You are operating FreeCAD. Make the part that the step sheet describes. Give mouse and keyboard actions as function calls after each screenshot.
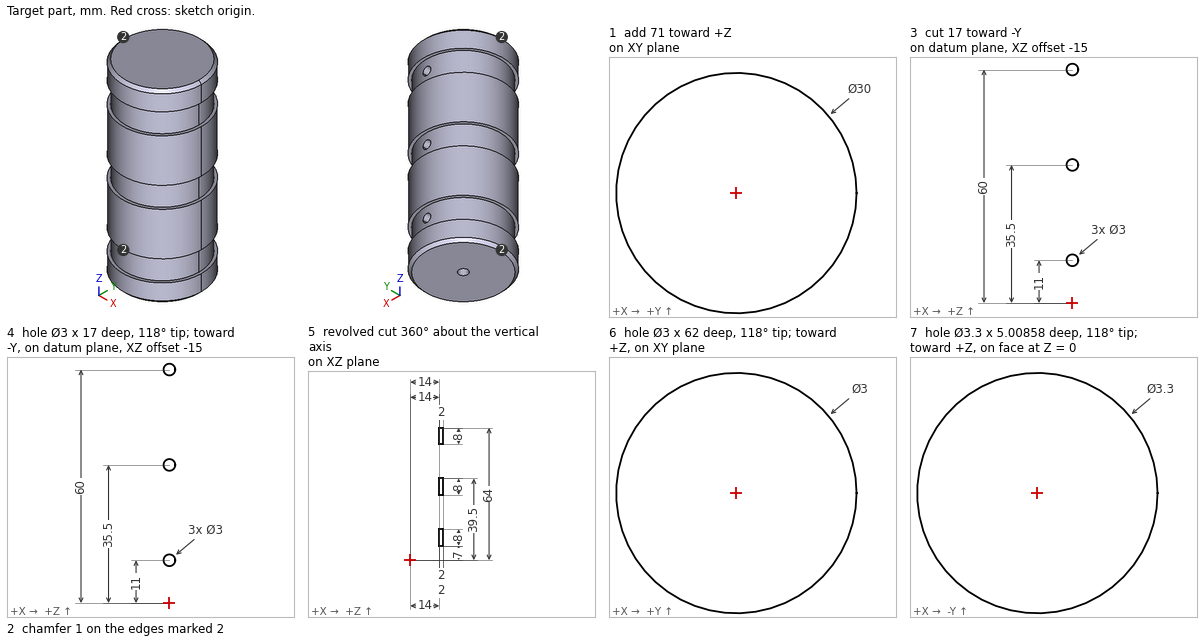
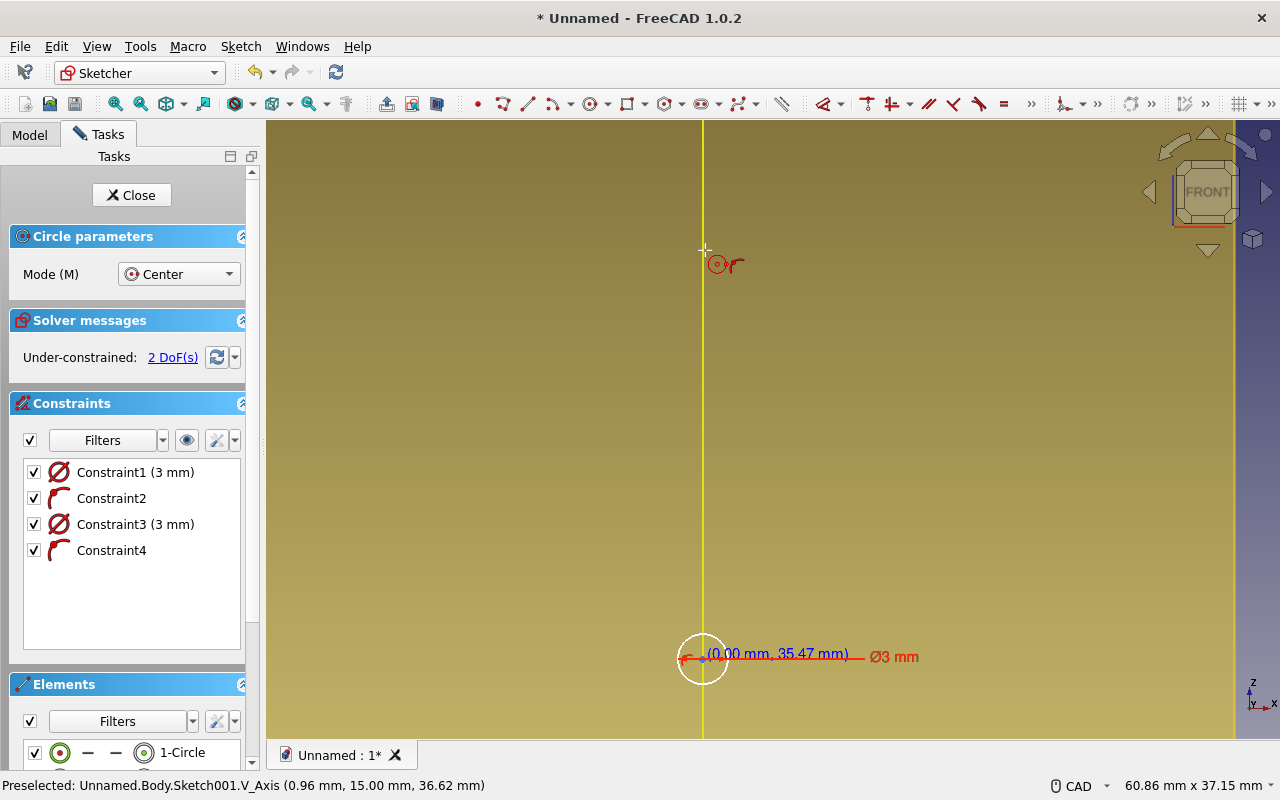
click(703, 250)
move(721, 233)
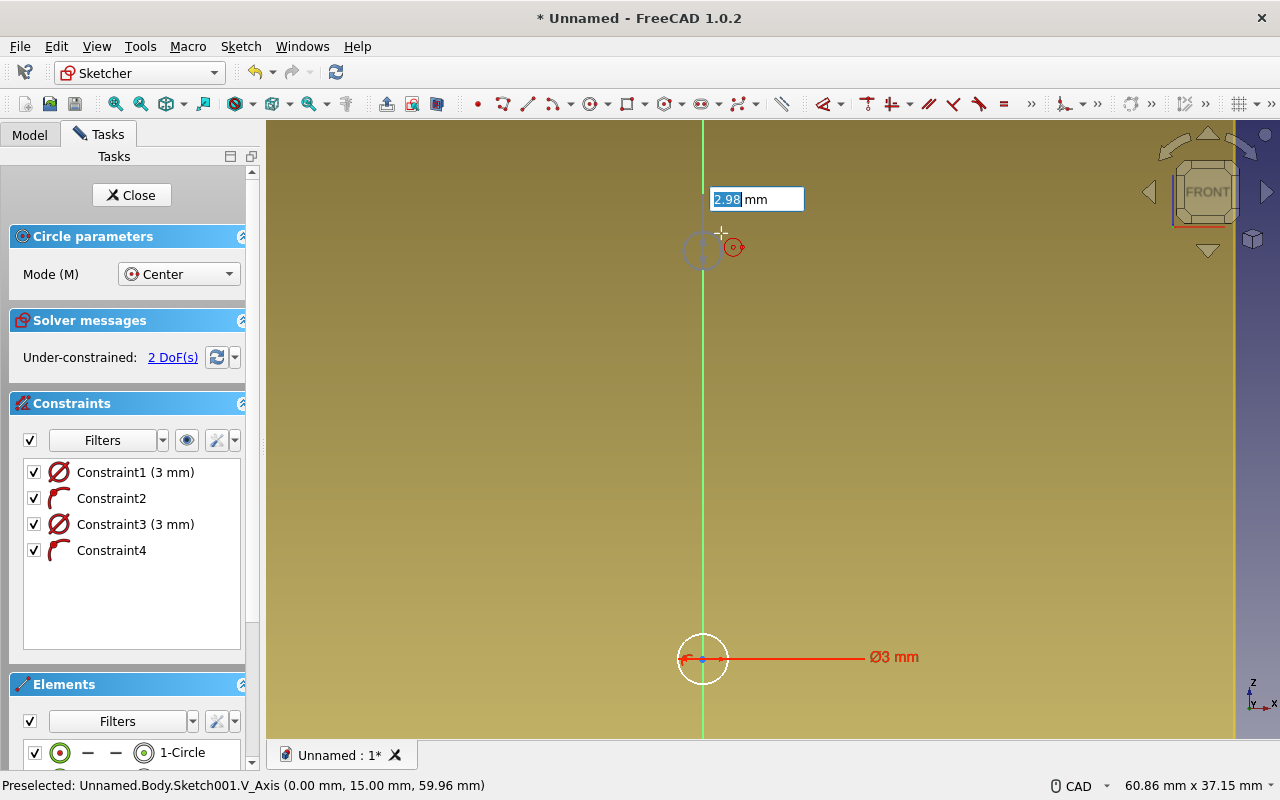
text(3)
key(Return)
key(Escape)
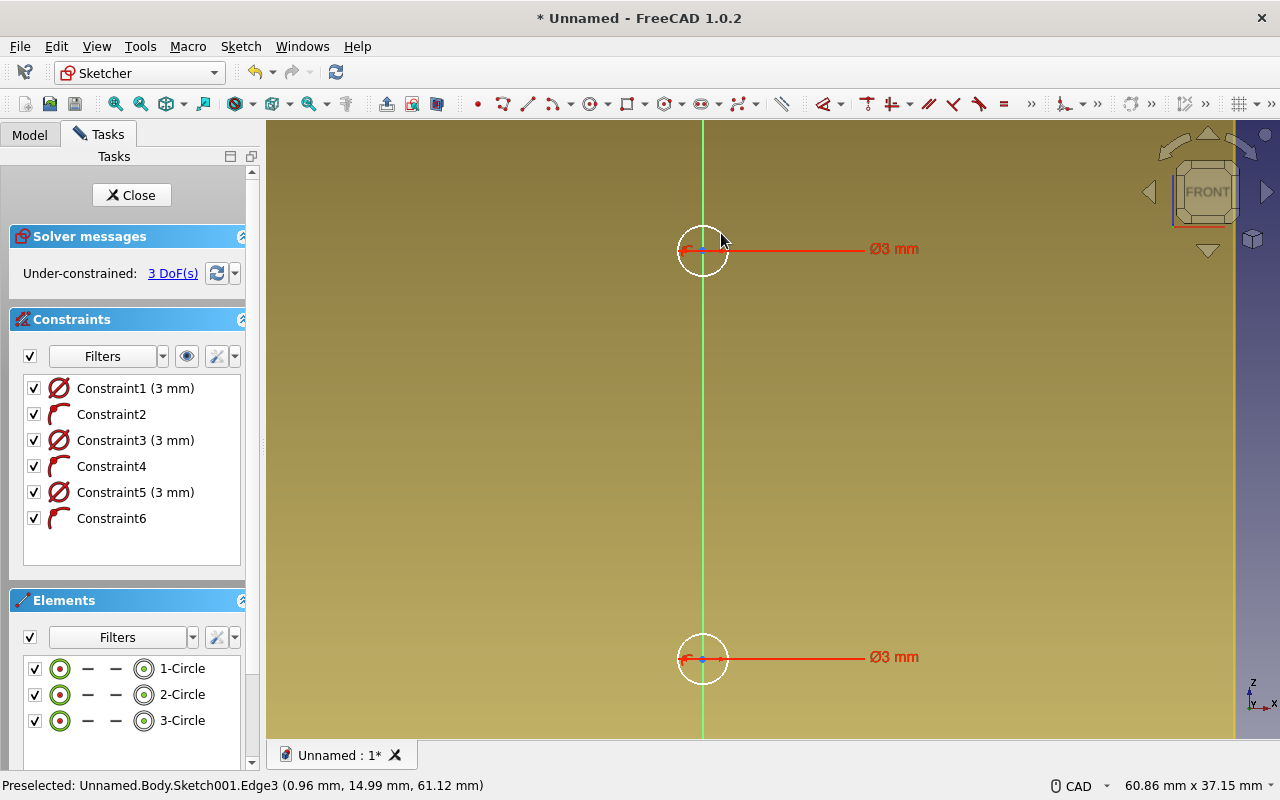
click(822, 104)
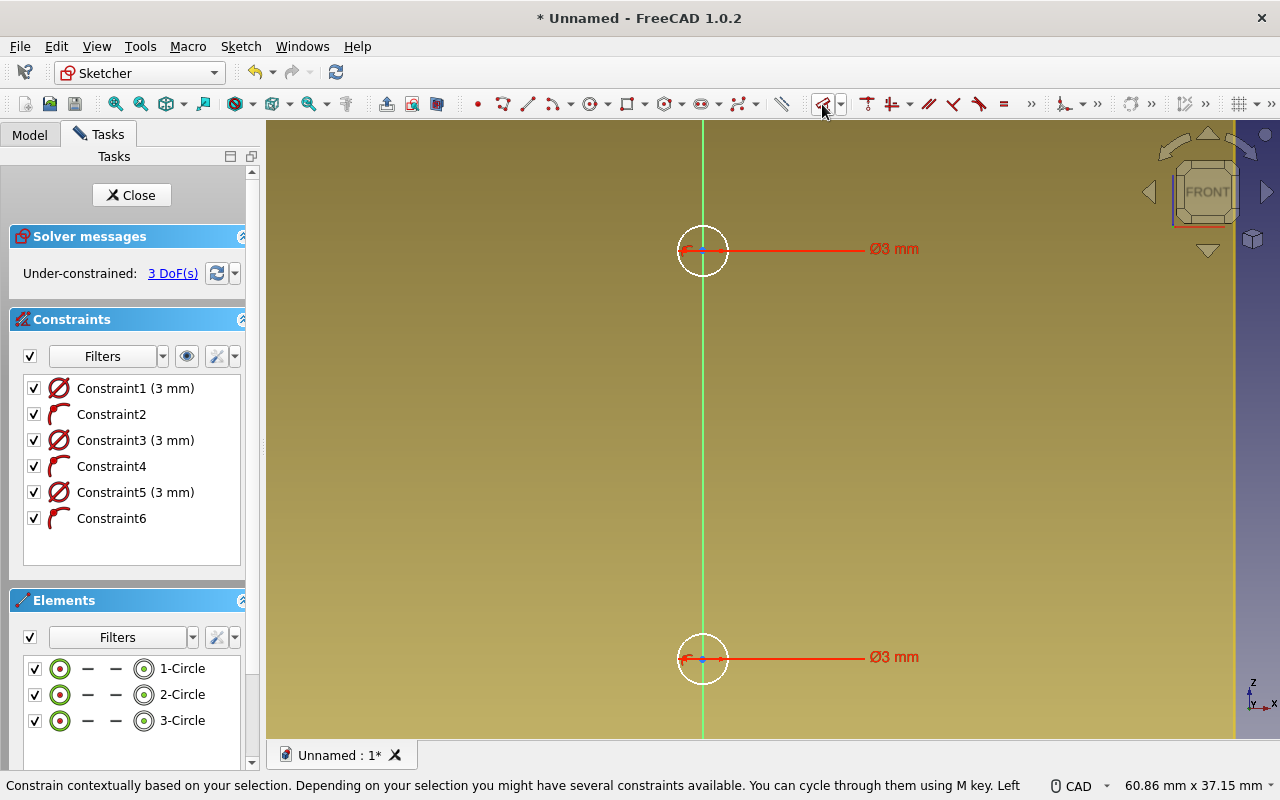
scroll(705, 250, down, 5)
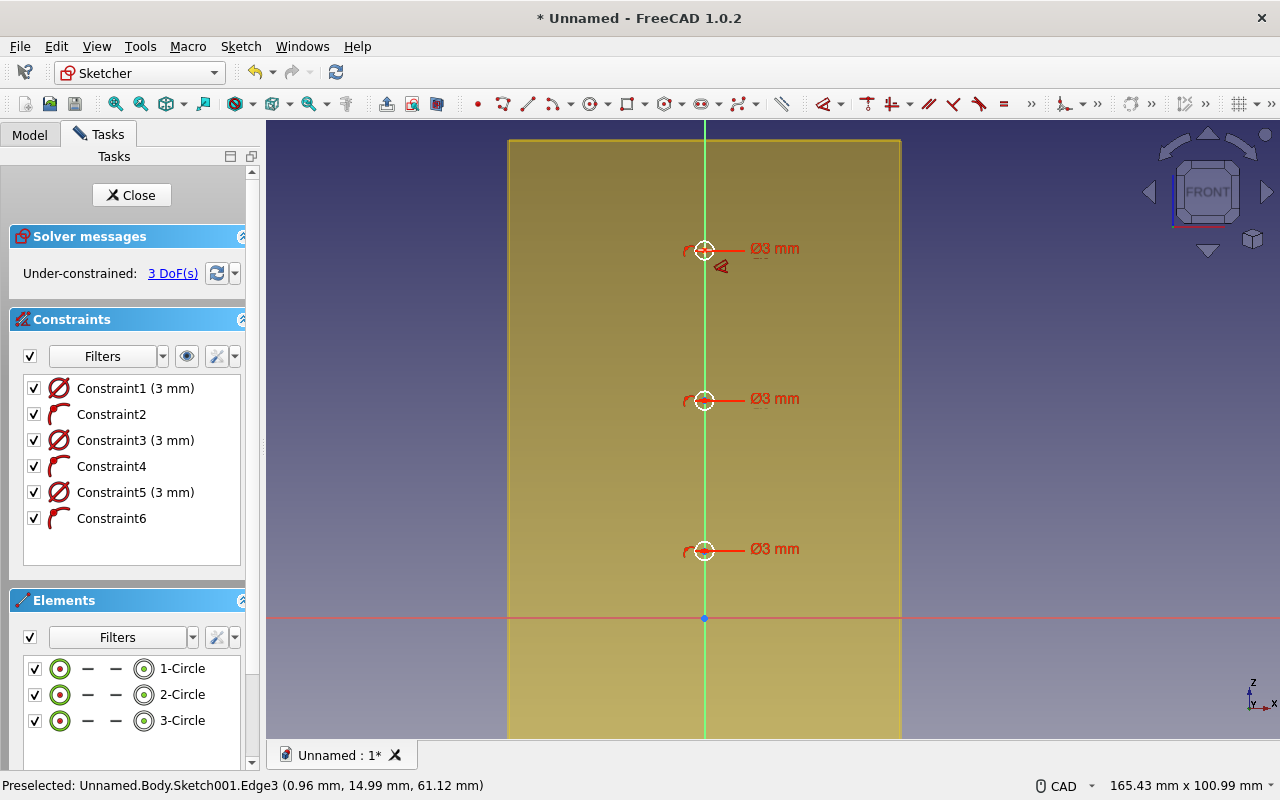
click(705, 551)
click(739, 585)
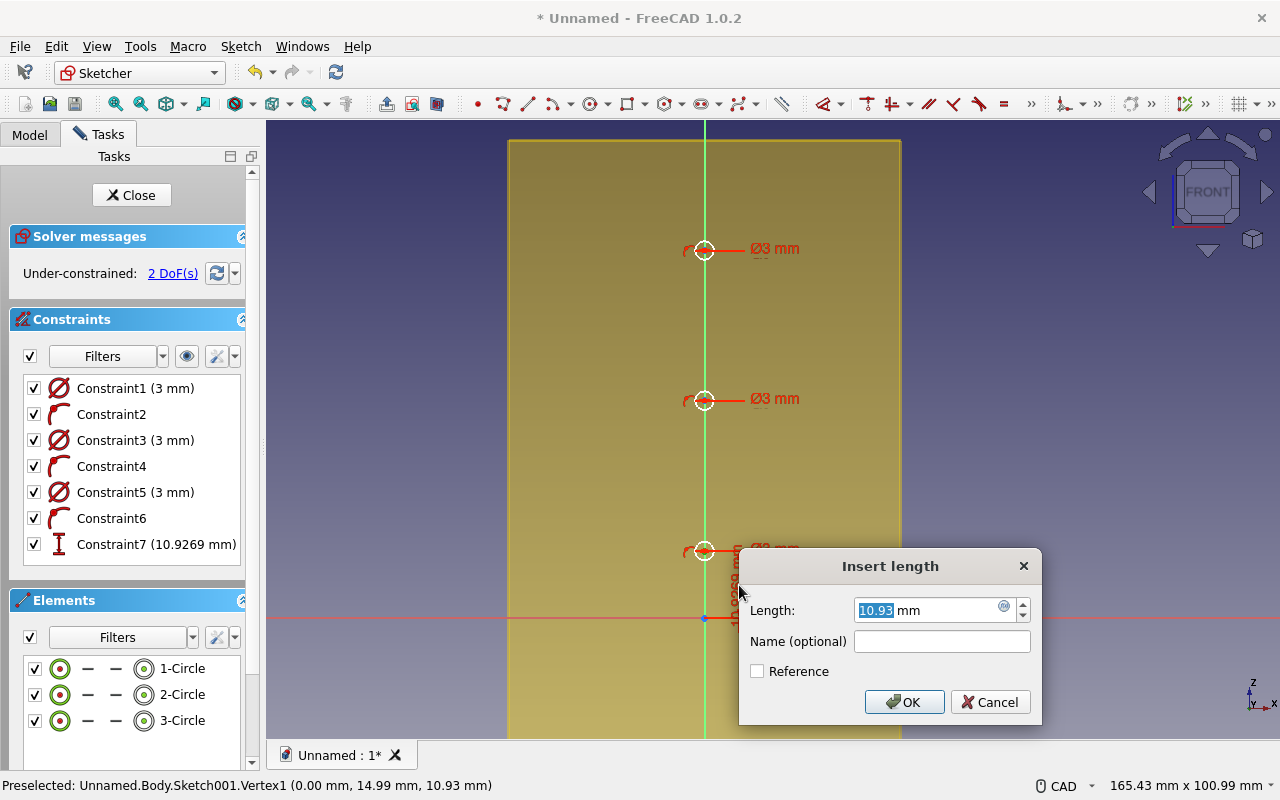
text(11)
key(Return)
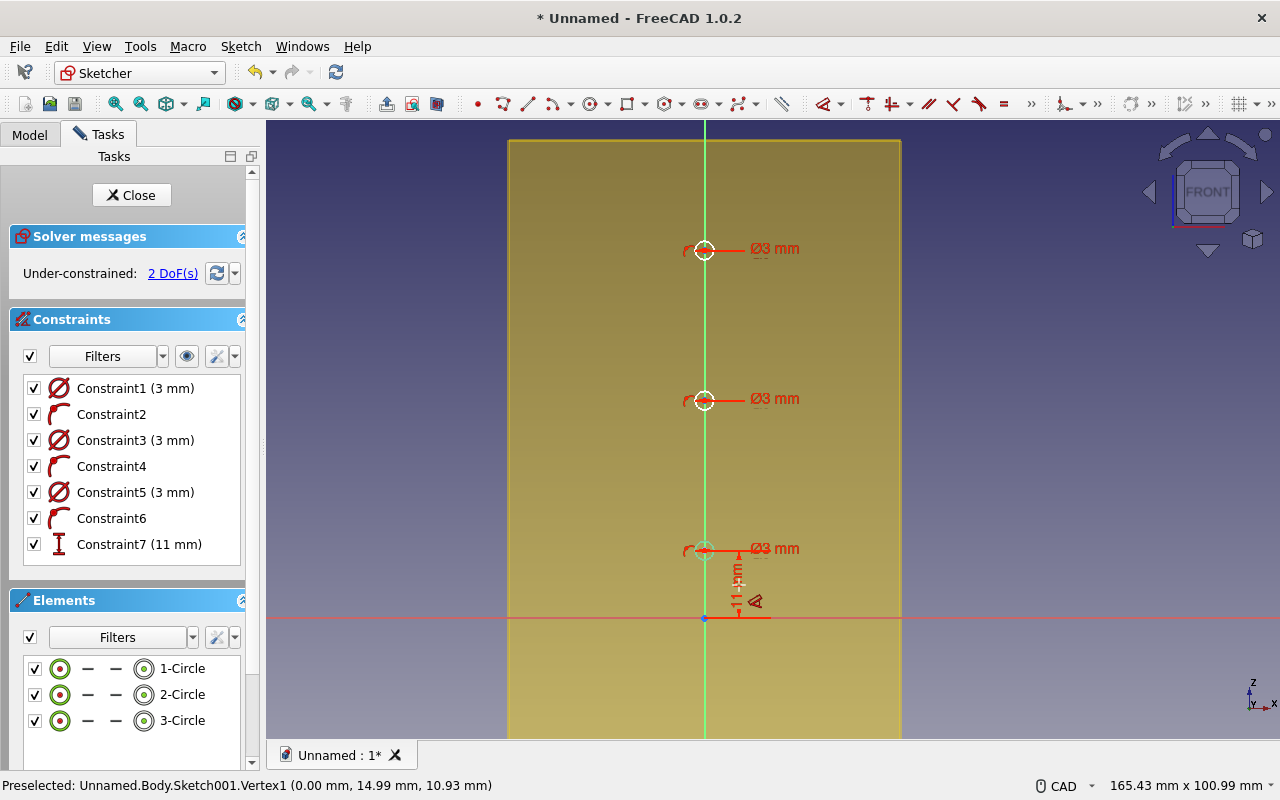
click(705, 251)
click(739, 434)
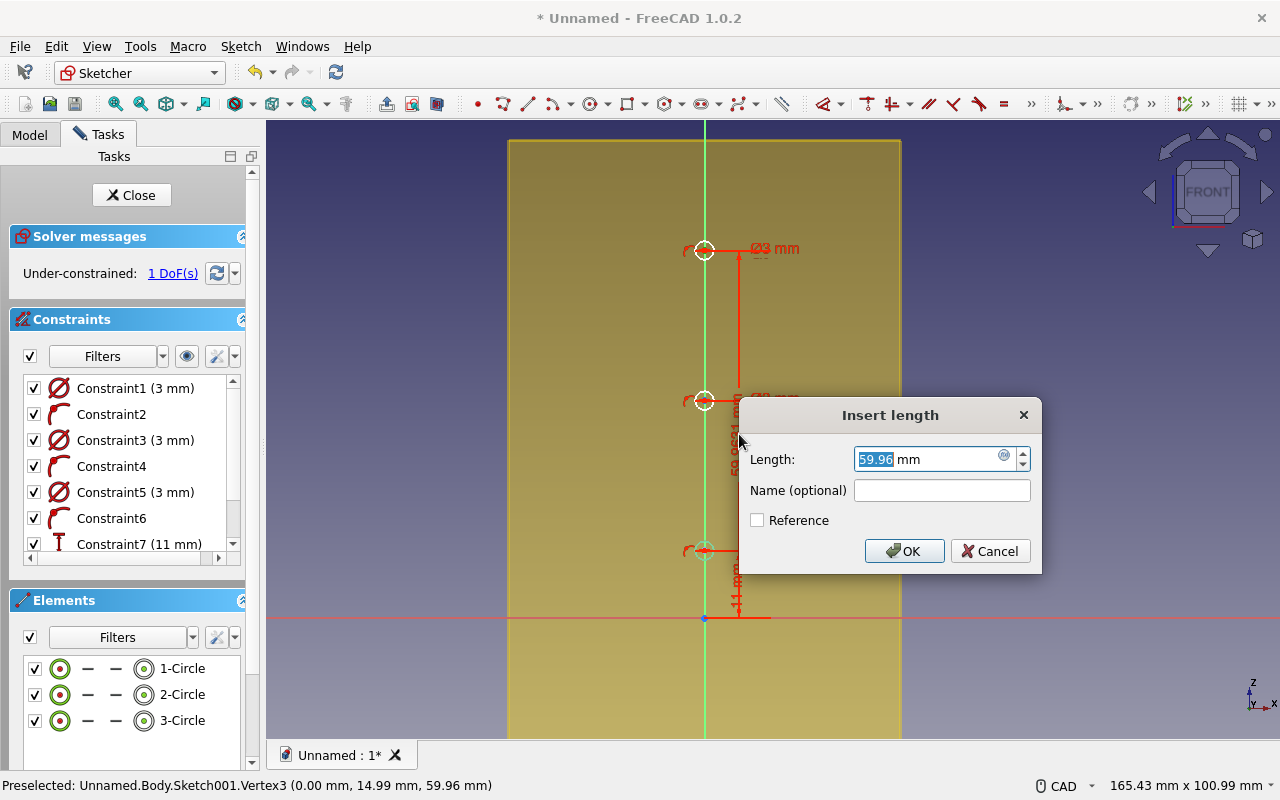
text(60)
key(Return)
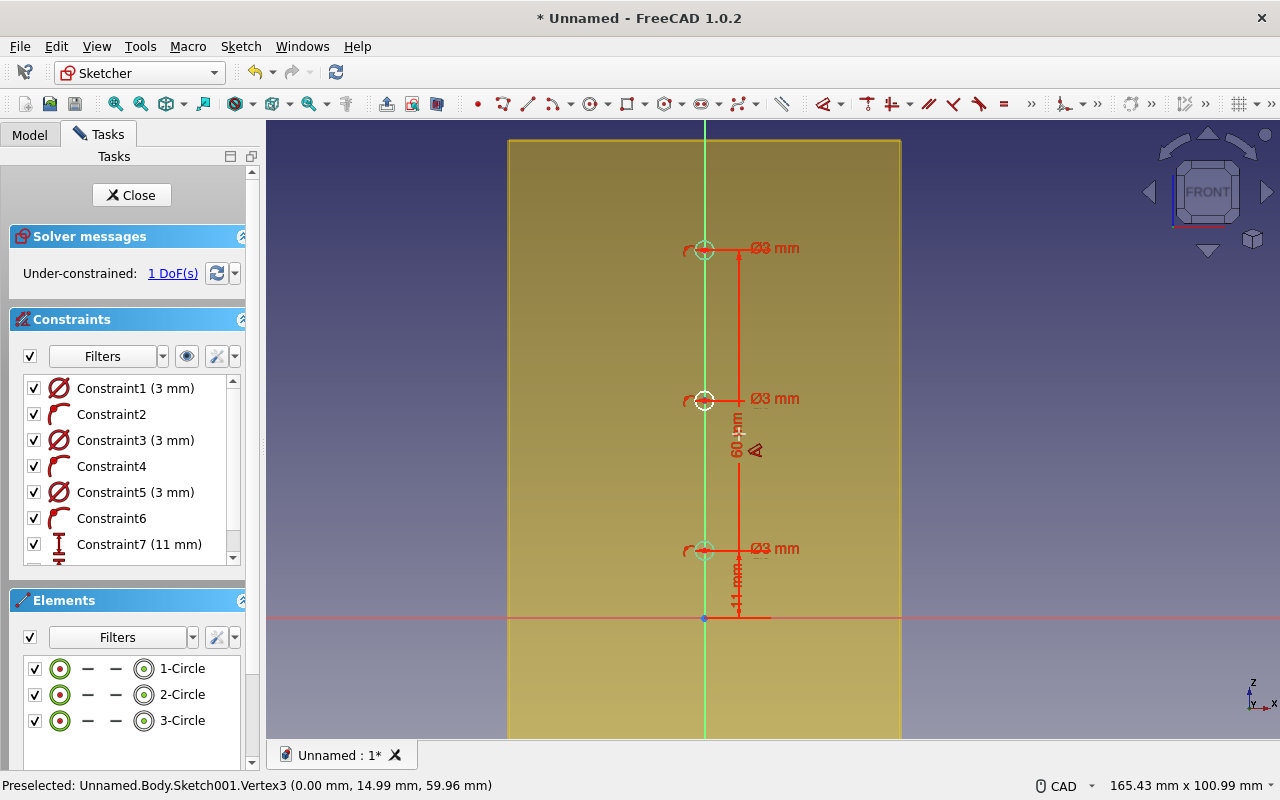
click(705, 401)
click(739, 509)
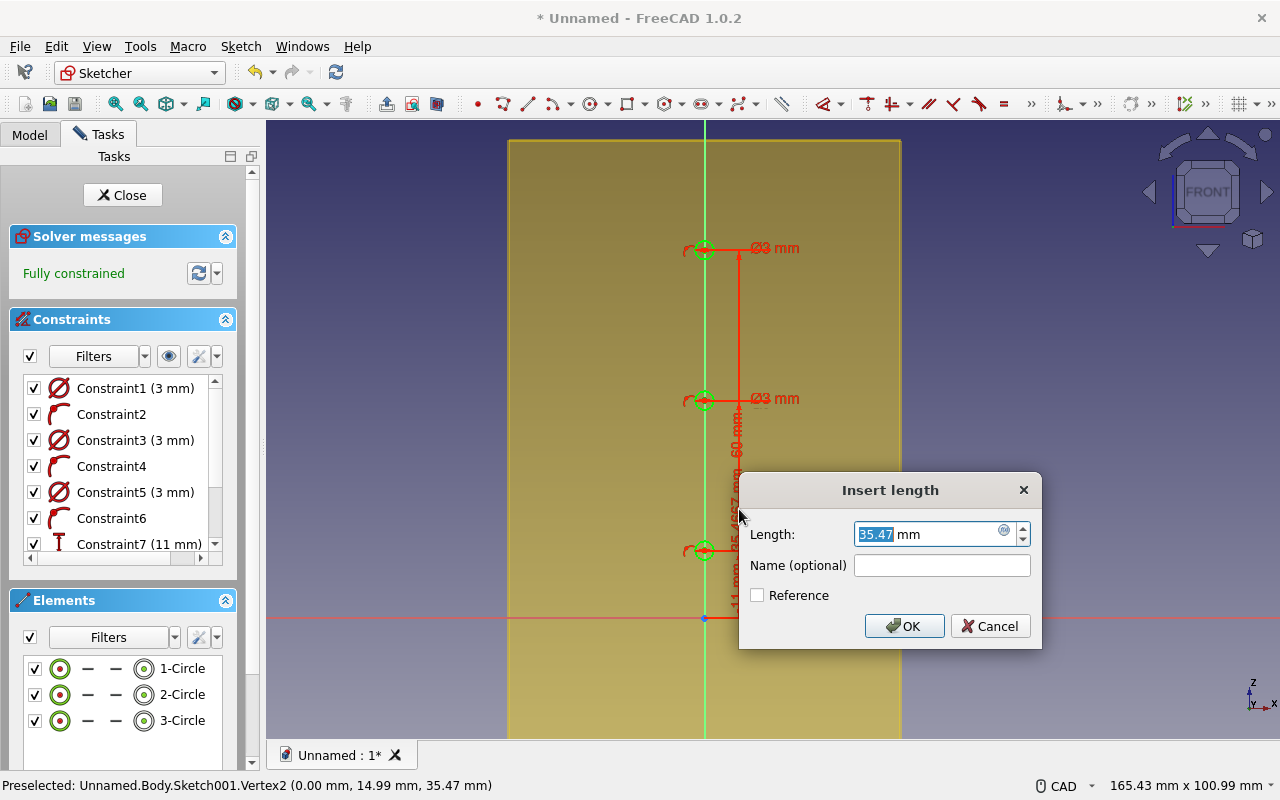
text(35.5)
key(Return)
key(Escape)